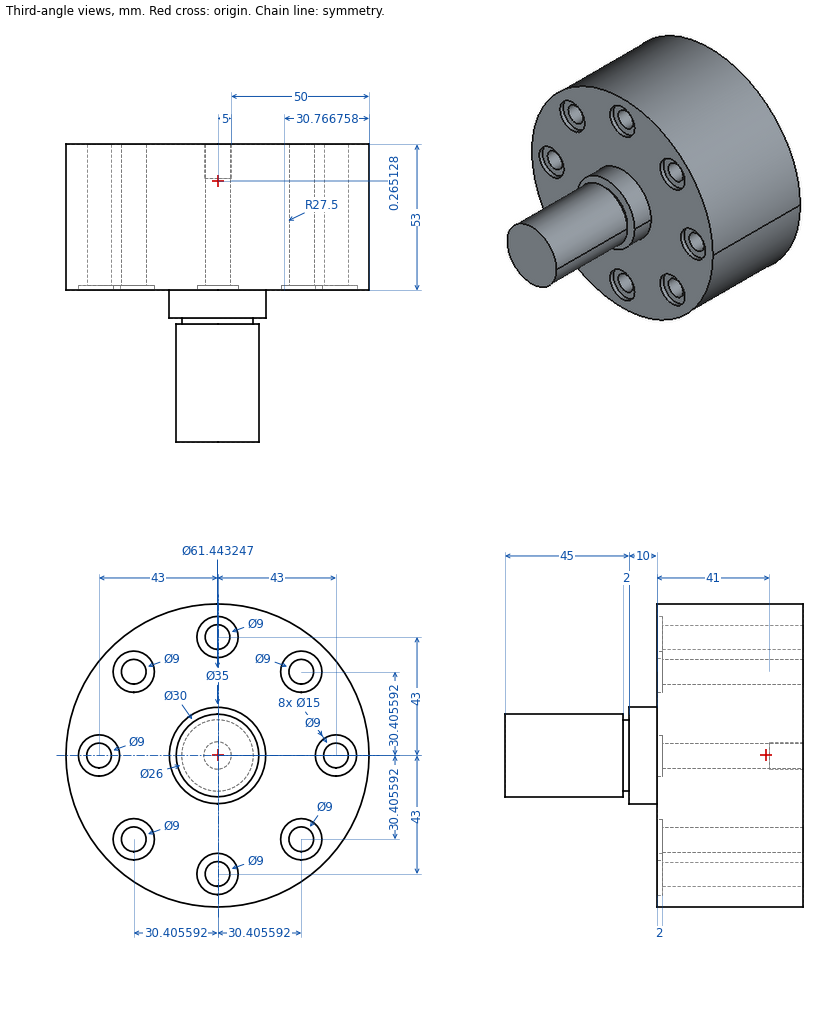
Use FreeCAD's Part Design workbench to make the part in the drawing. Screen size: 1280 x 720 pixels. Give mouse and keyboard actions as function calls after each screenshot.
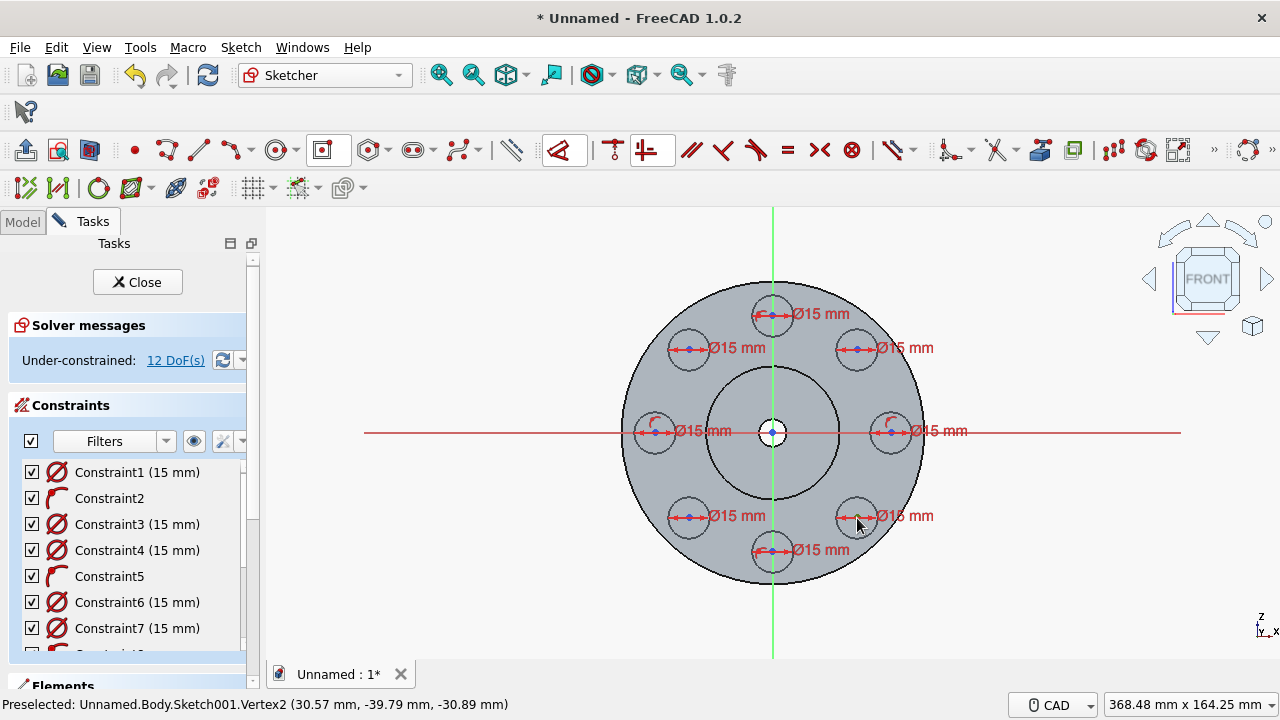
click(689, 518)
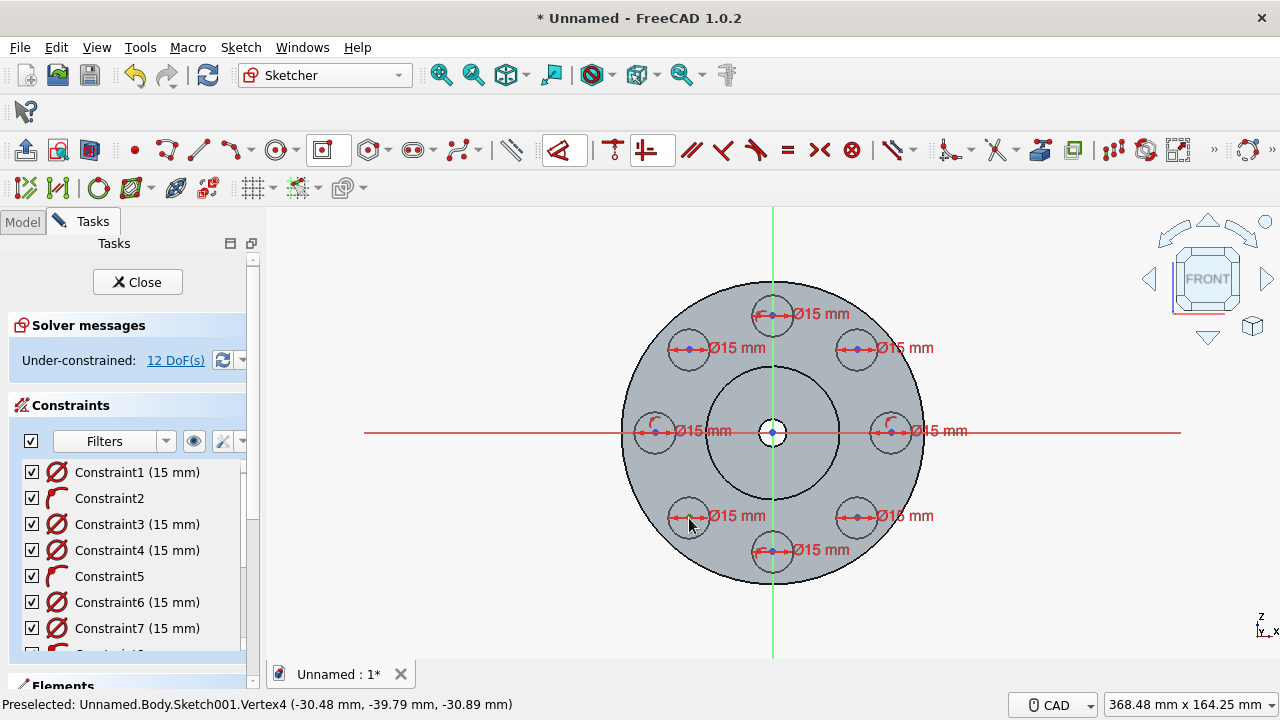
click(773, 603)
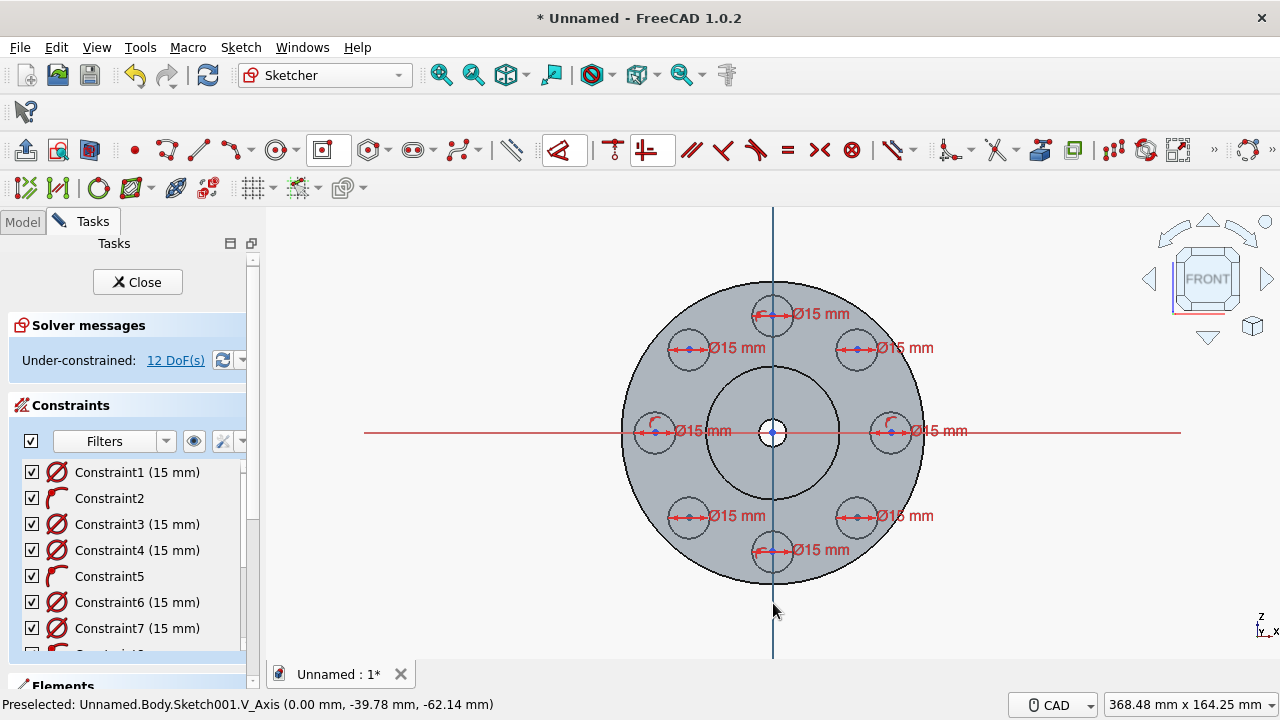
click(820, 150)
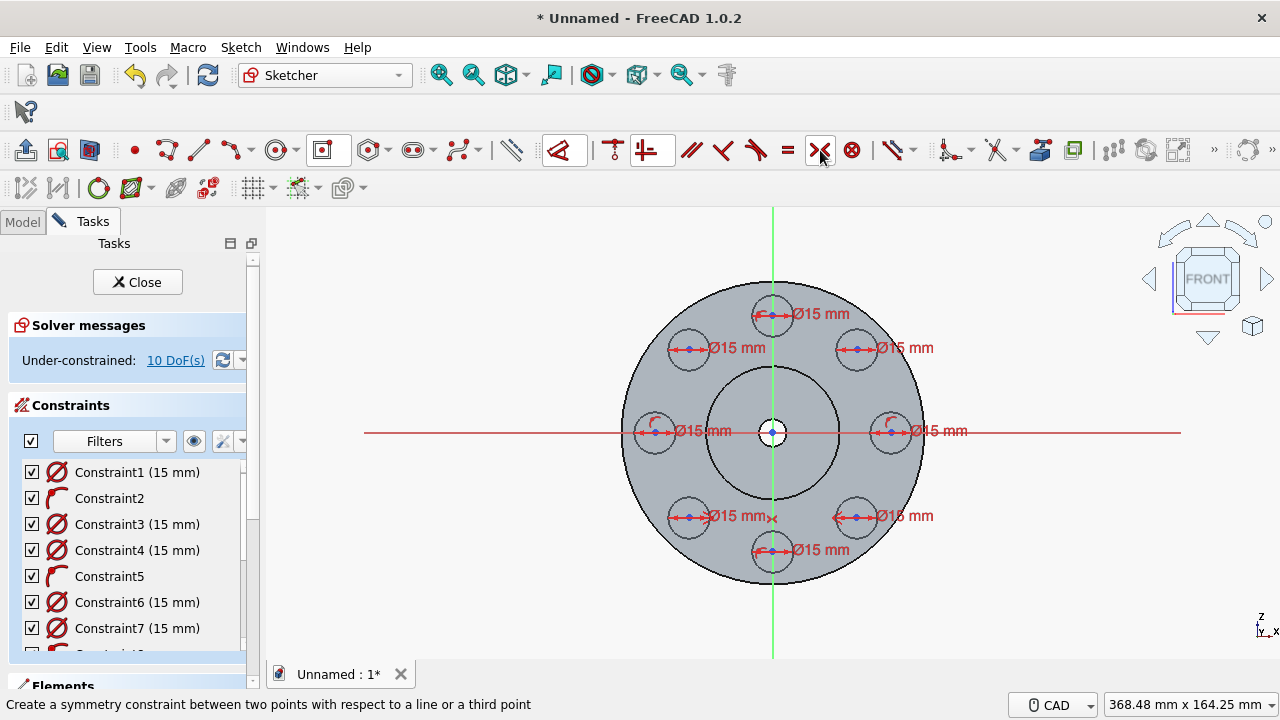
click(689, 518)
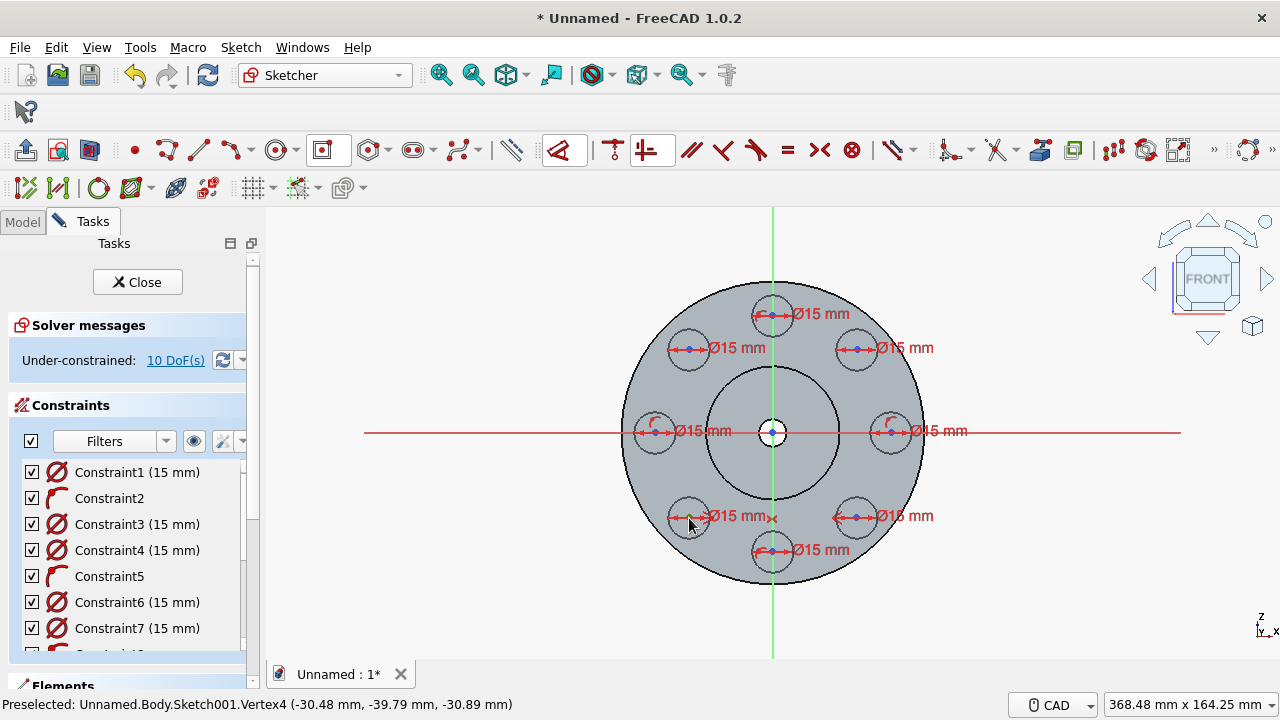
click(689, 350)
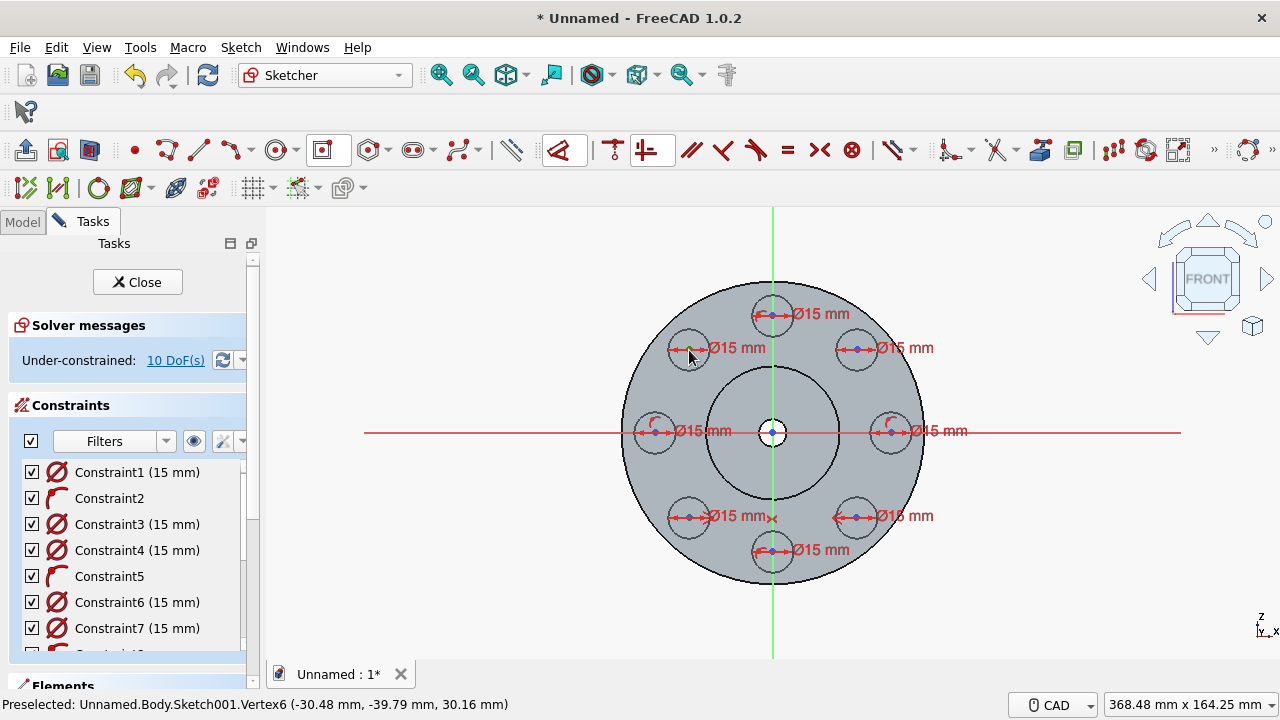
click(411, 433)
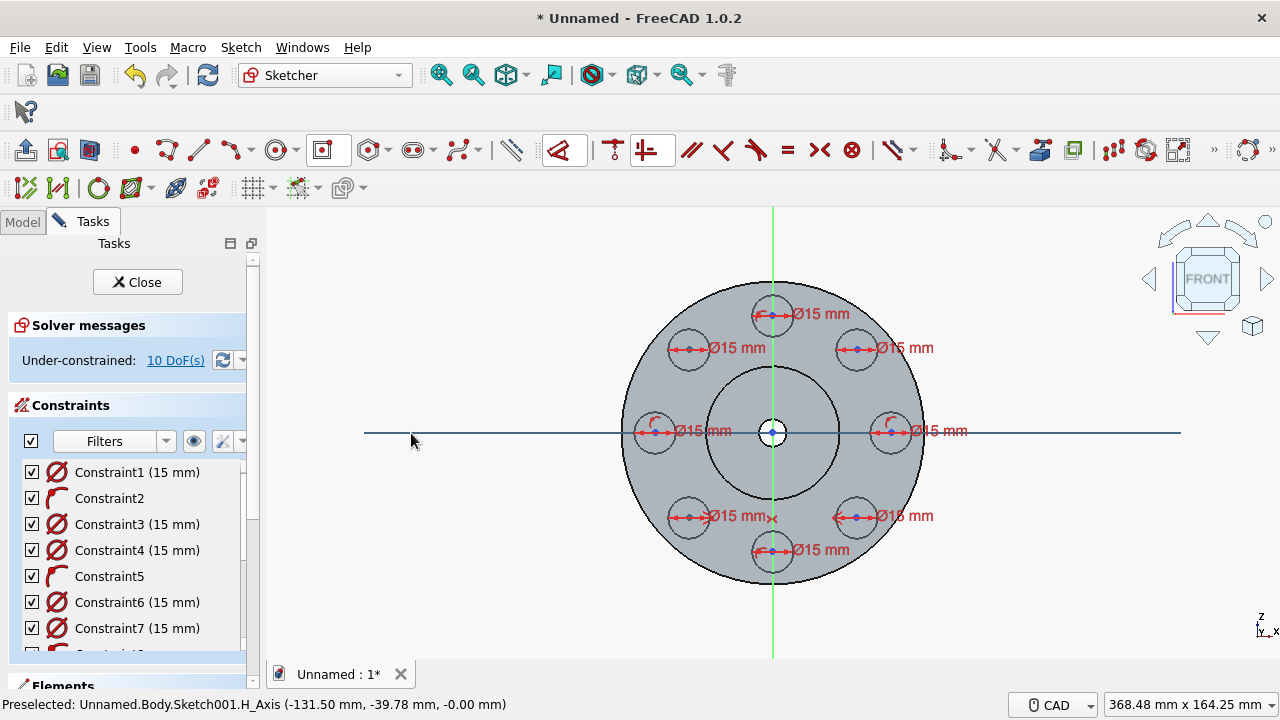
click(820, 150)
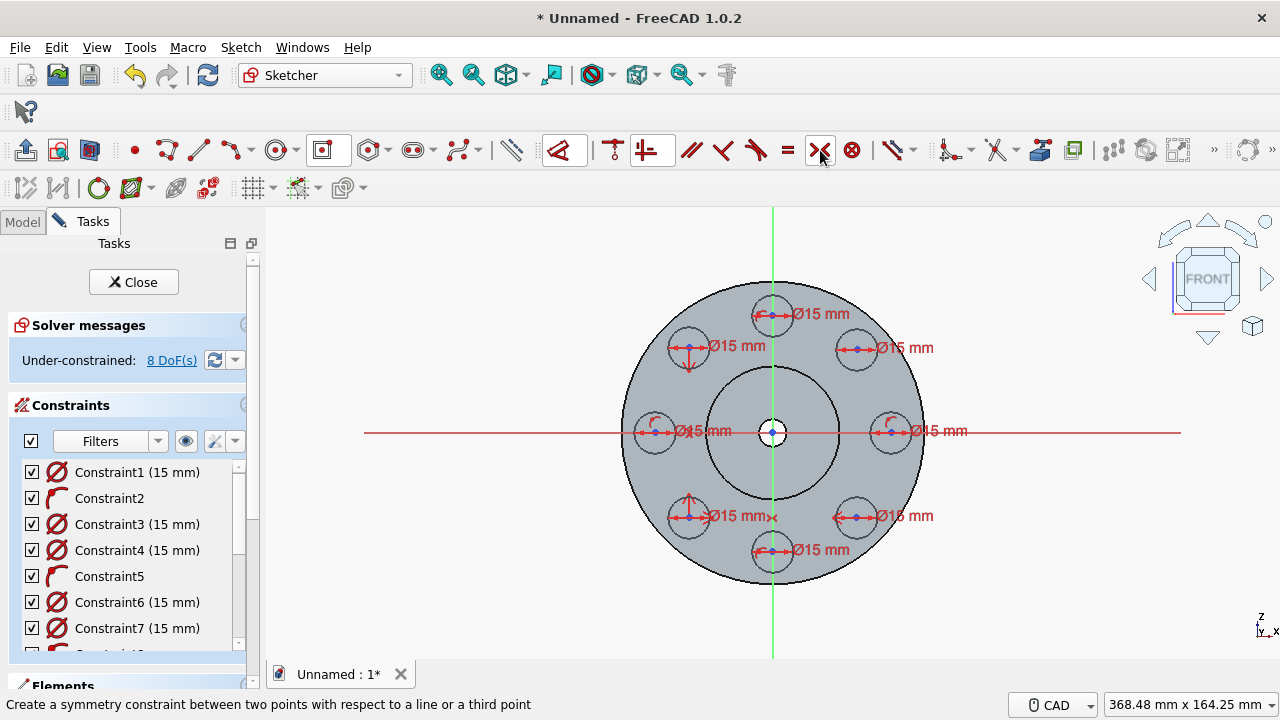
click(857, 518)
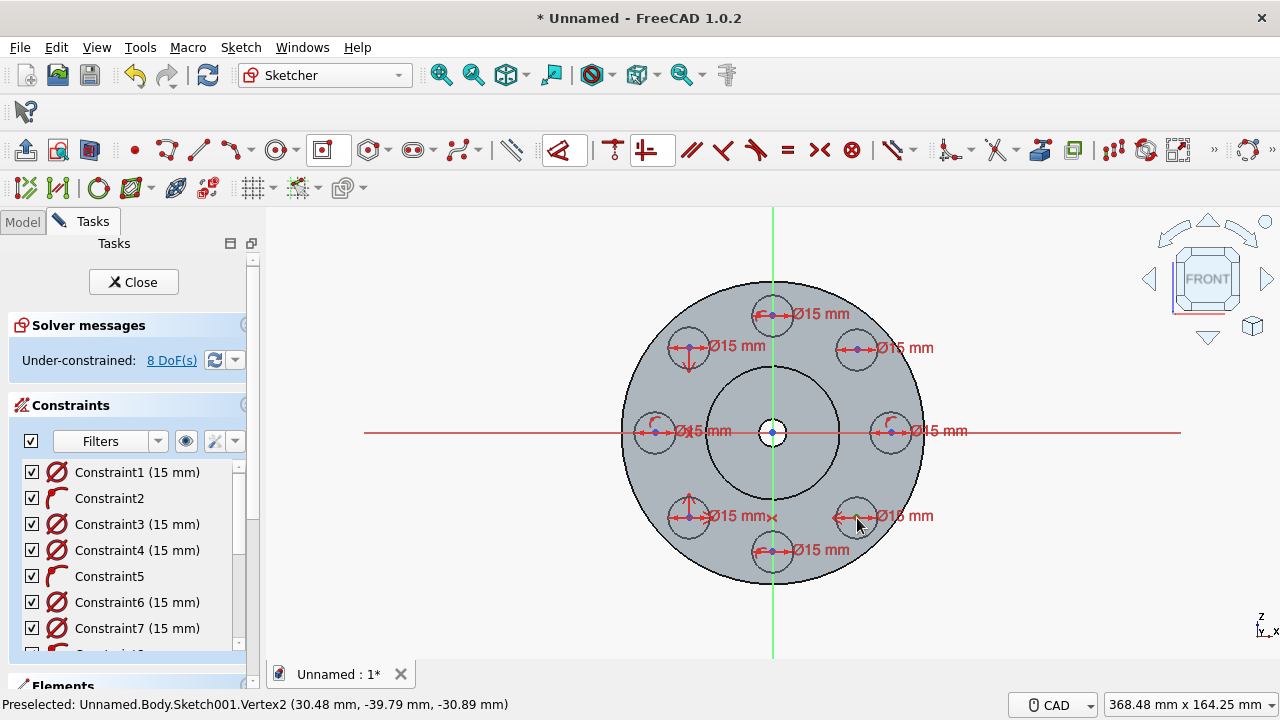
click(857, 350)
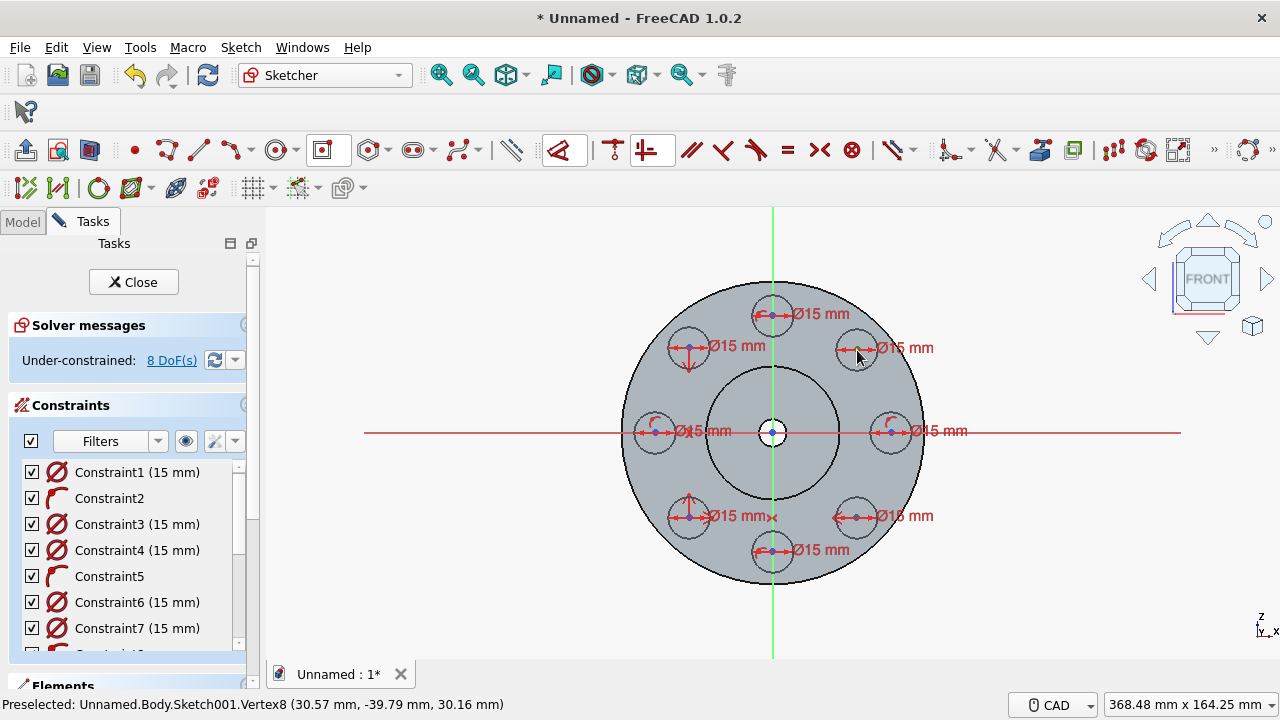
click(411, 433)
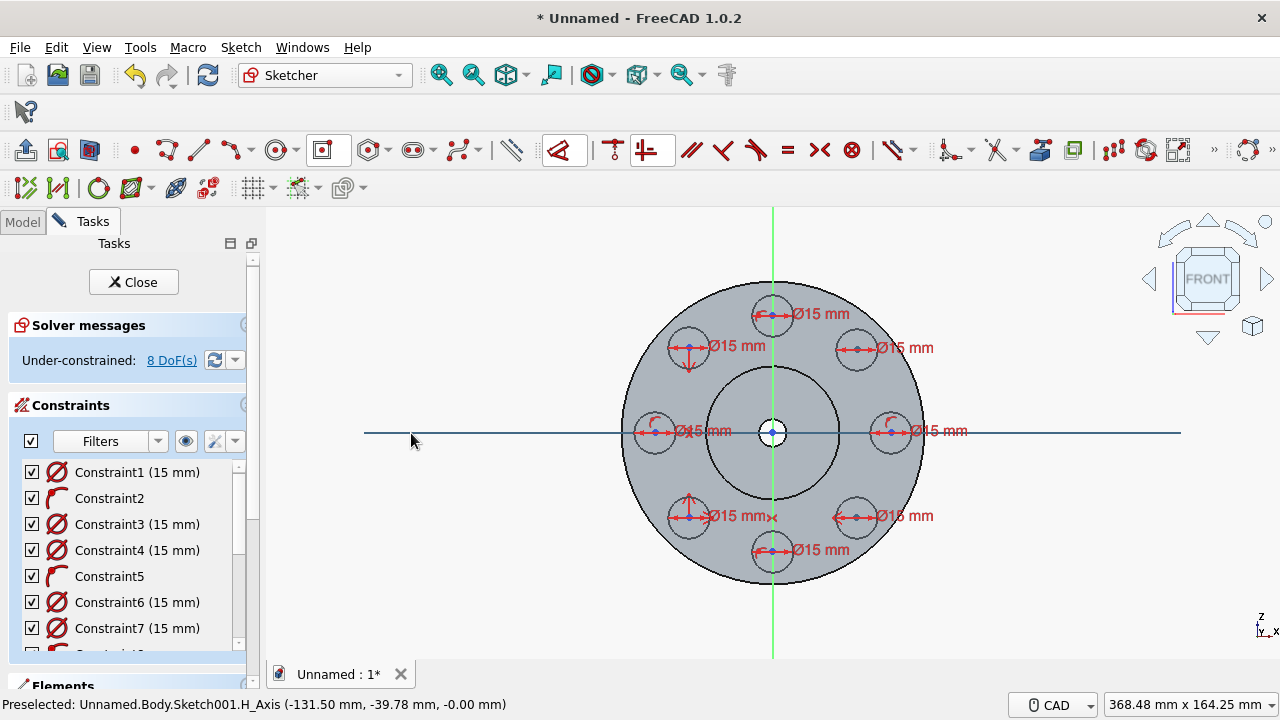
key(s)